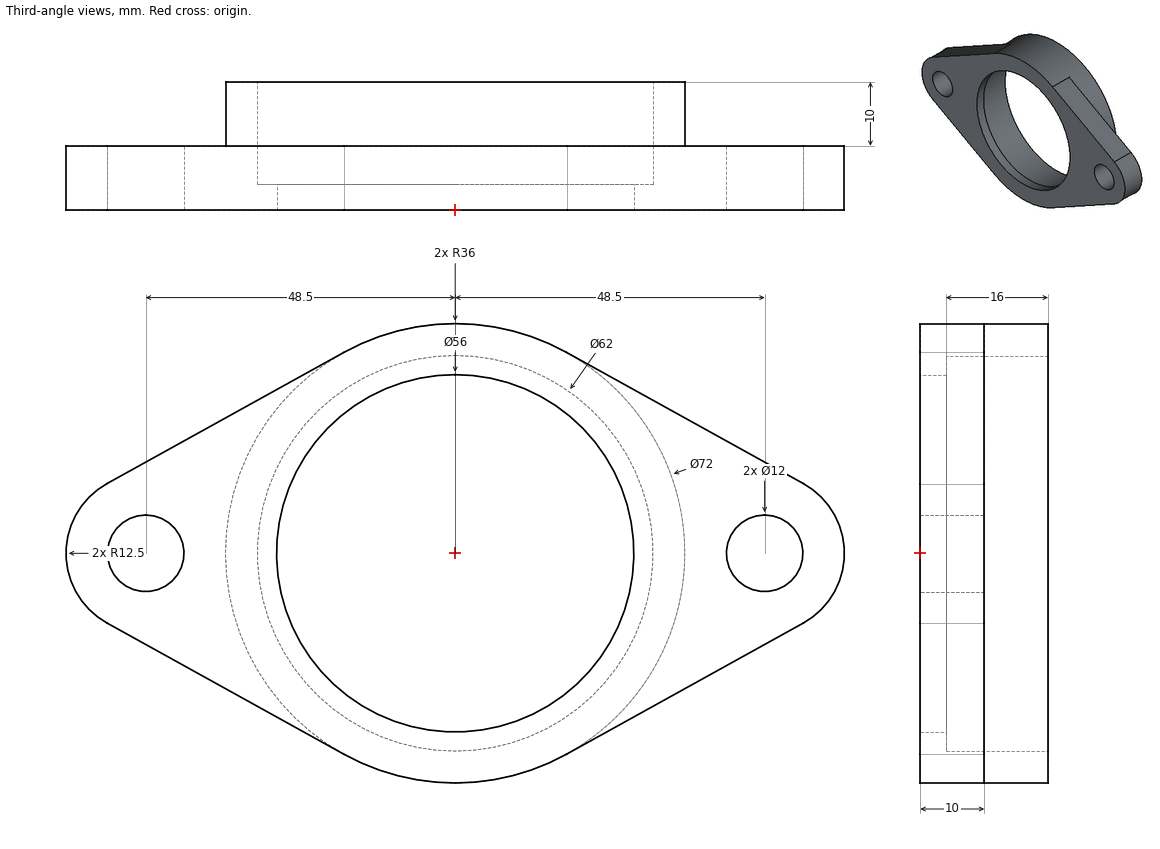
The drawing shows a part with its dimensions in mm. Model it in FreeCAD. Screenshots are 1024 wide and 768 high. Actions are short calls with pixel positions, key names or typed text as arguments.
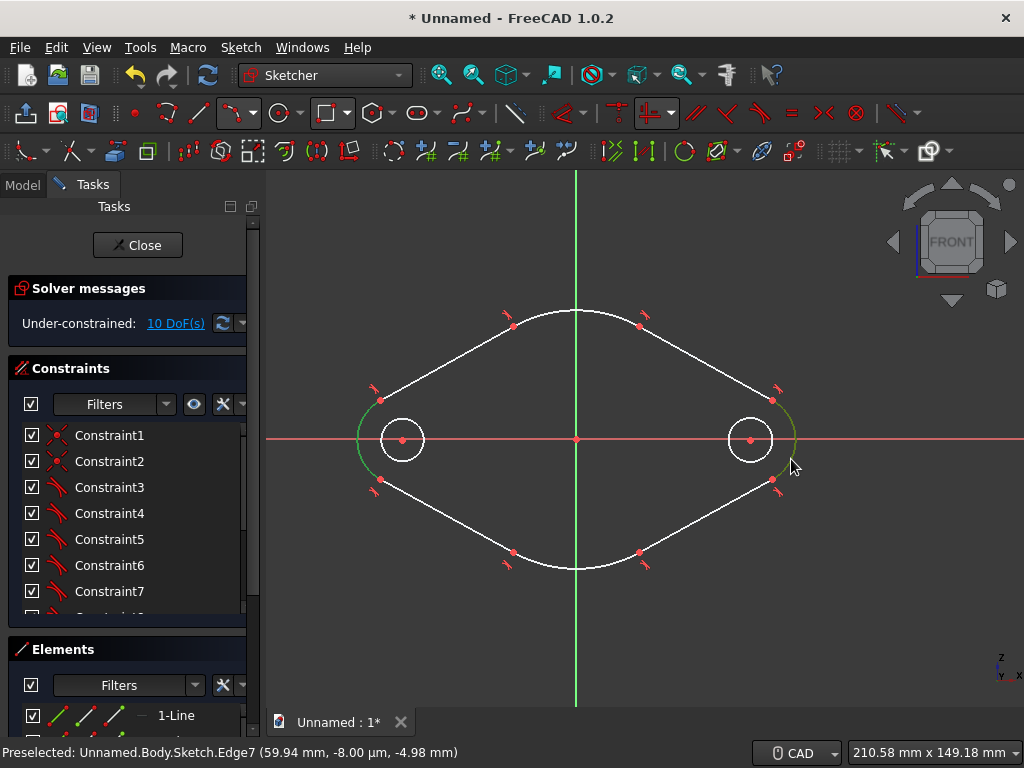
click(792, 114)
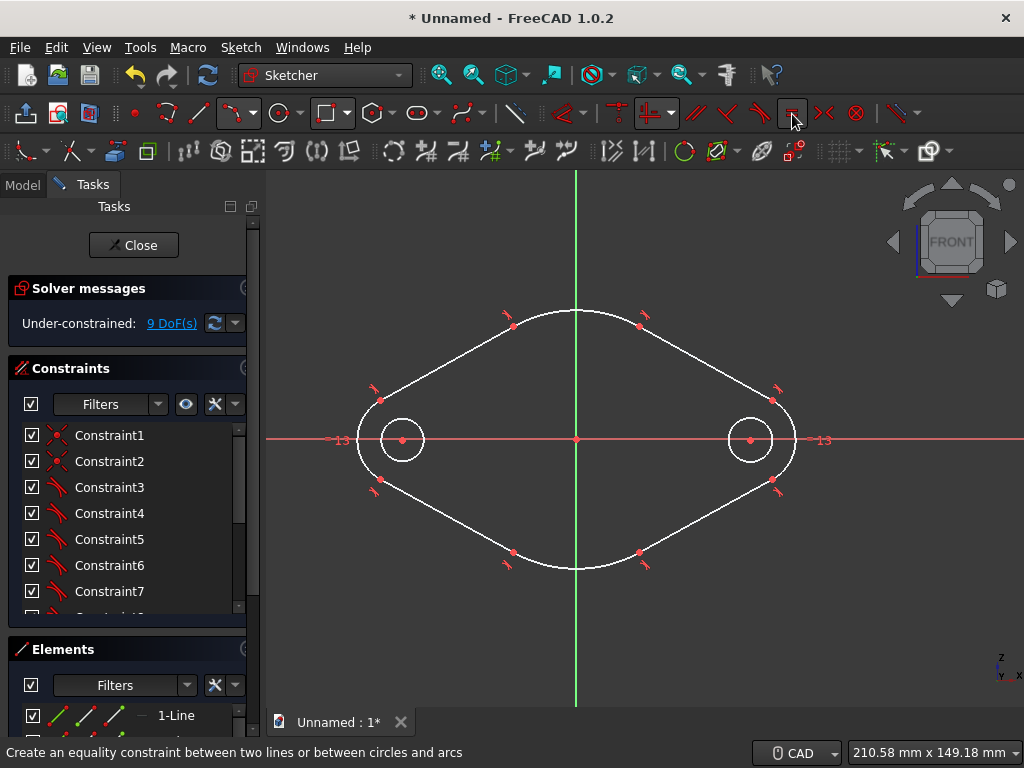
click(602, 313)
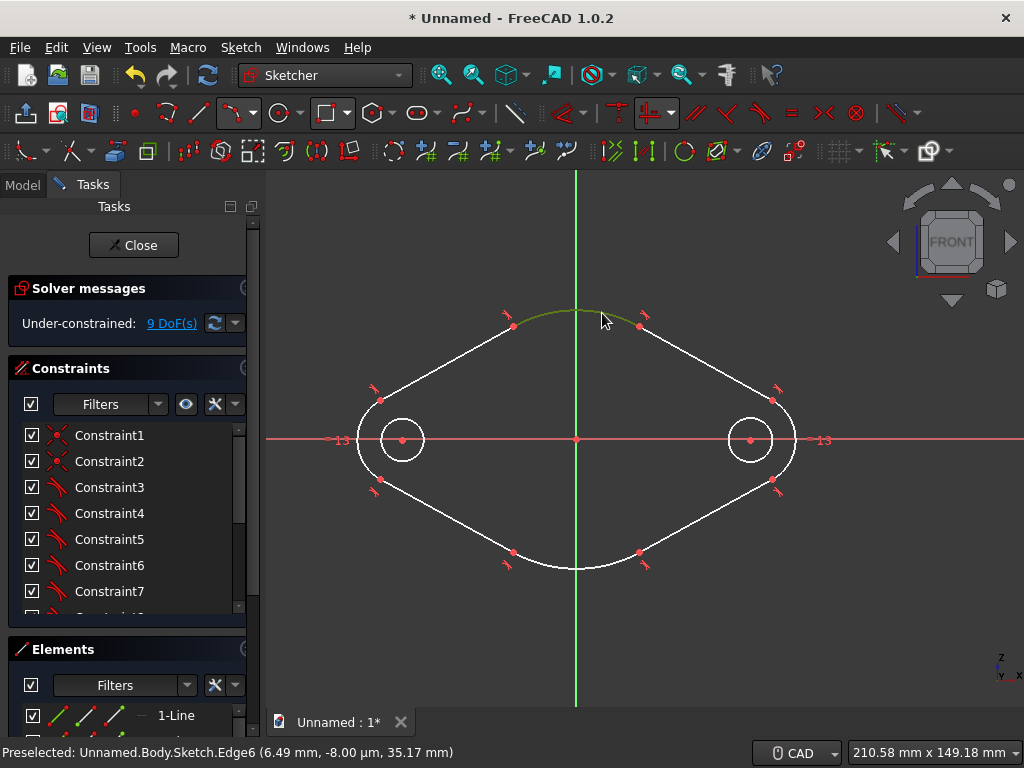
click(551, 566)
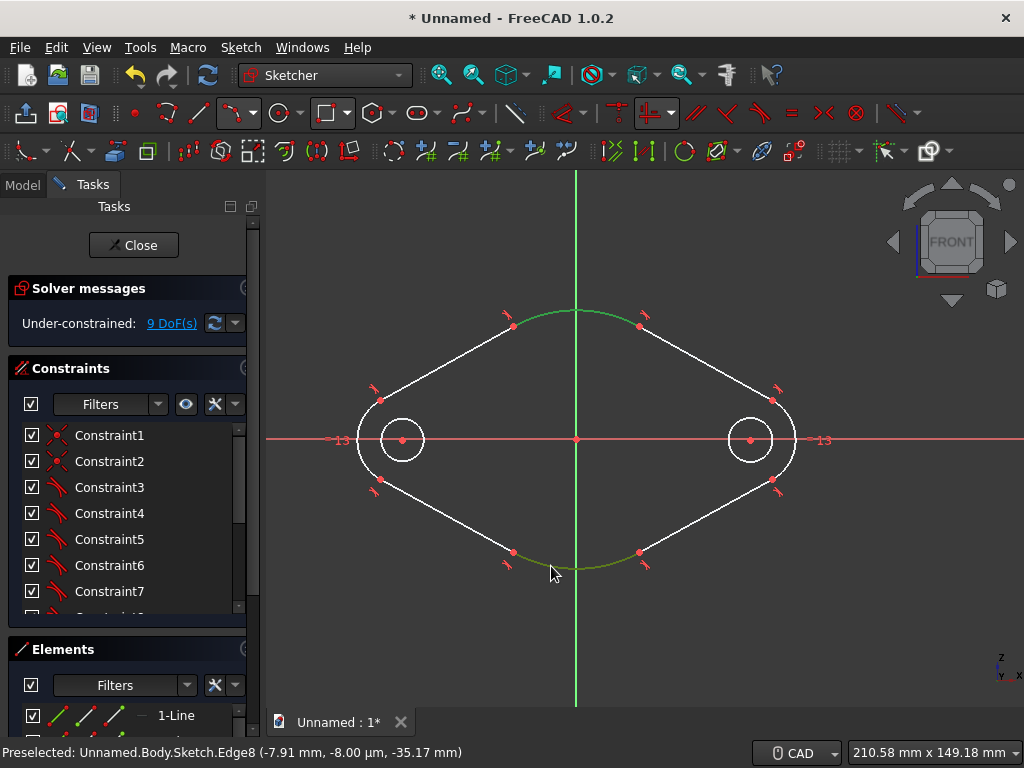
click(792, 114)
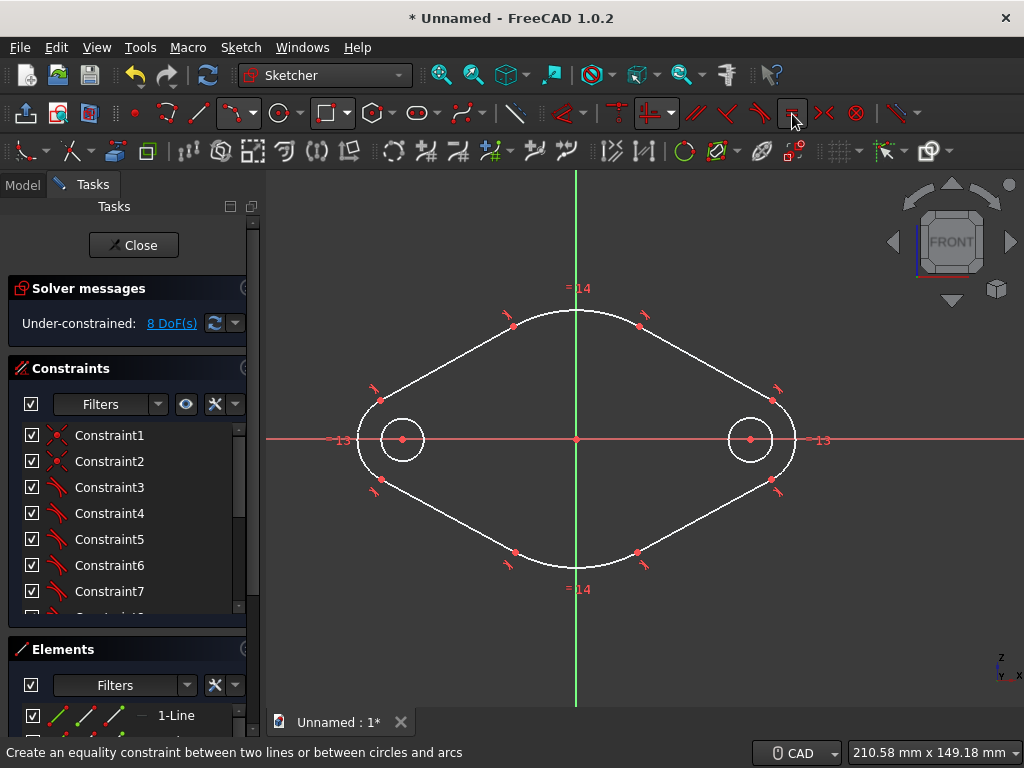
click(766, 424)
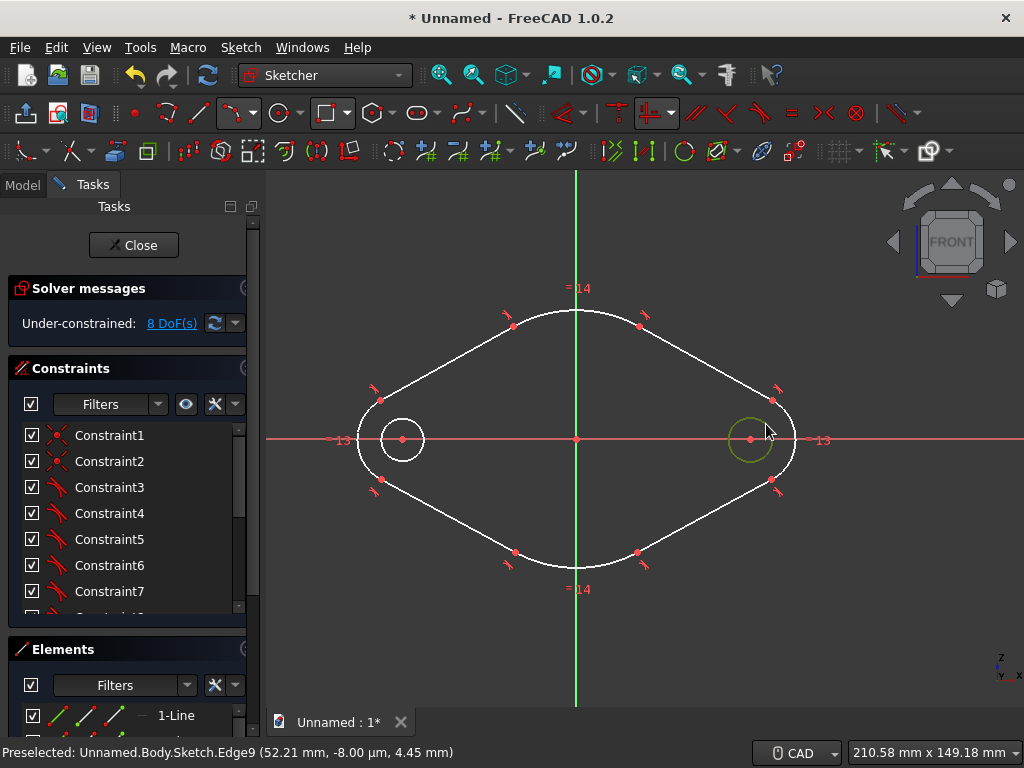
click(417, 425)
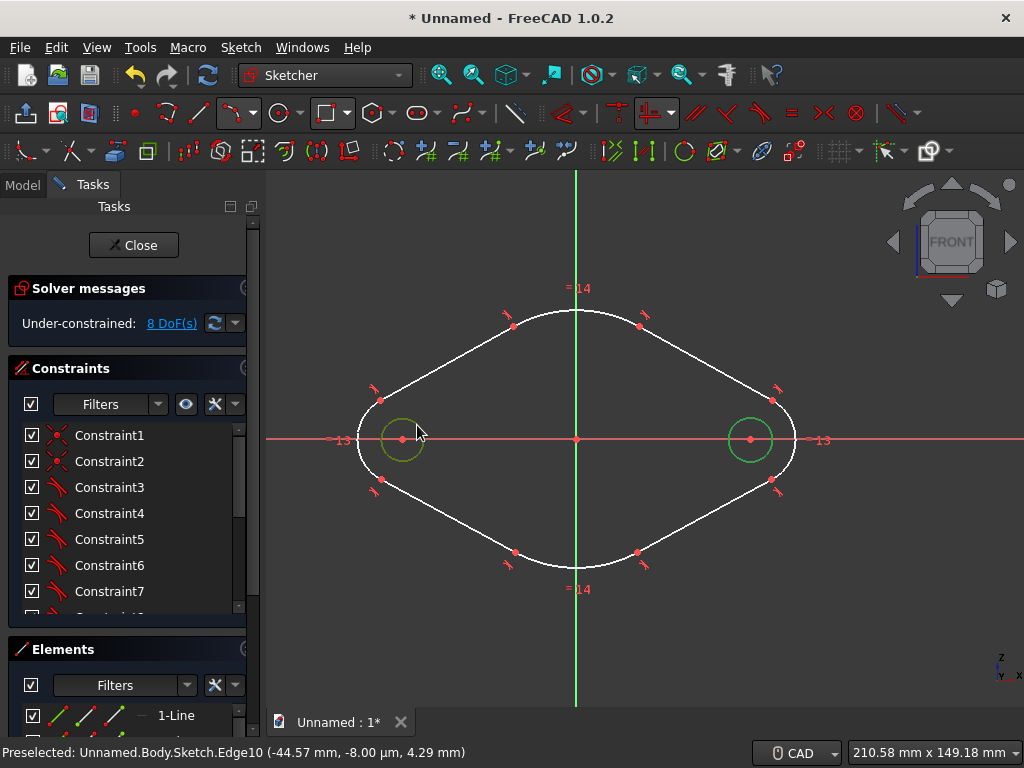
click(792, 114)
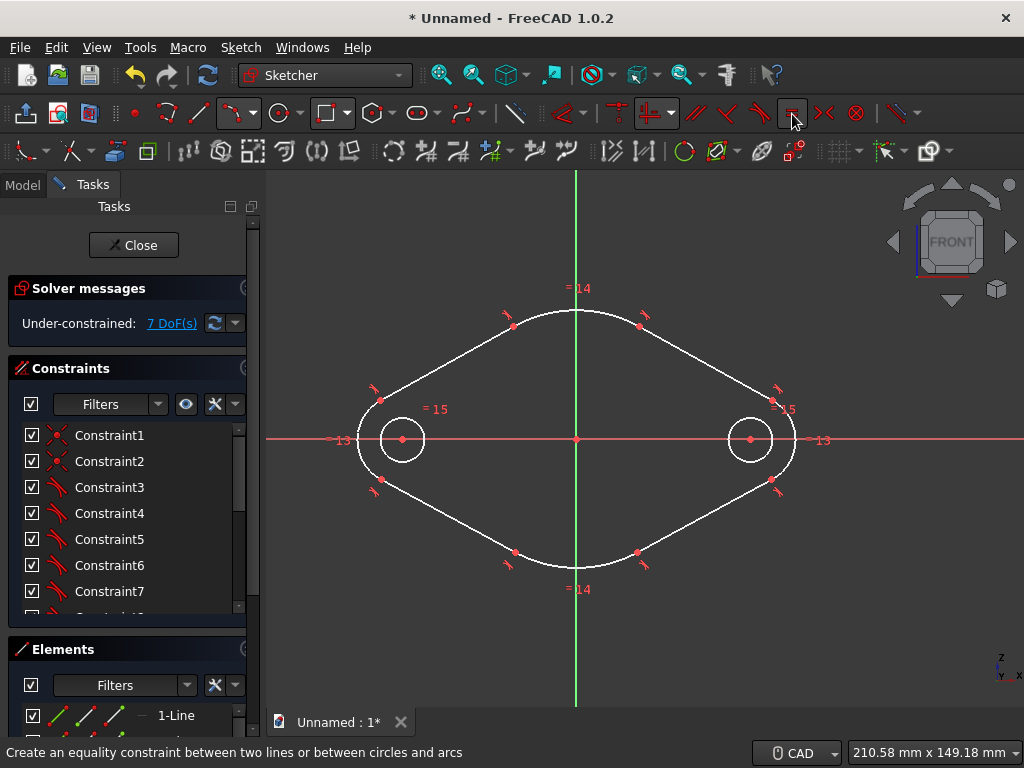
click(403, 440)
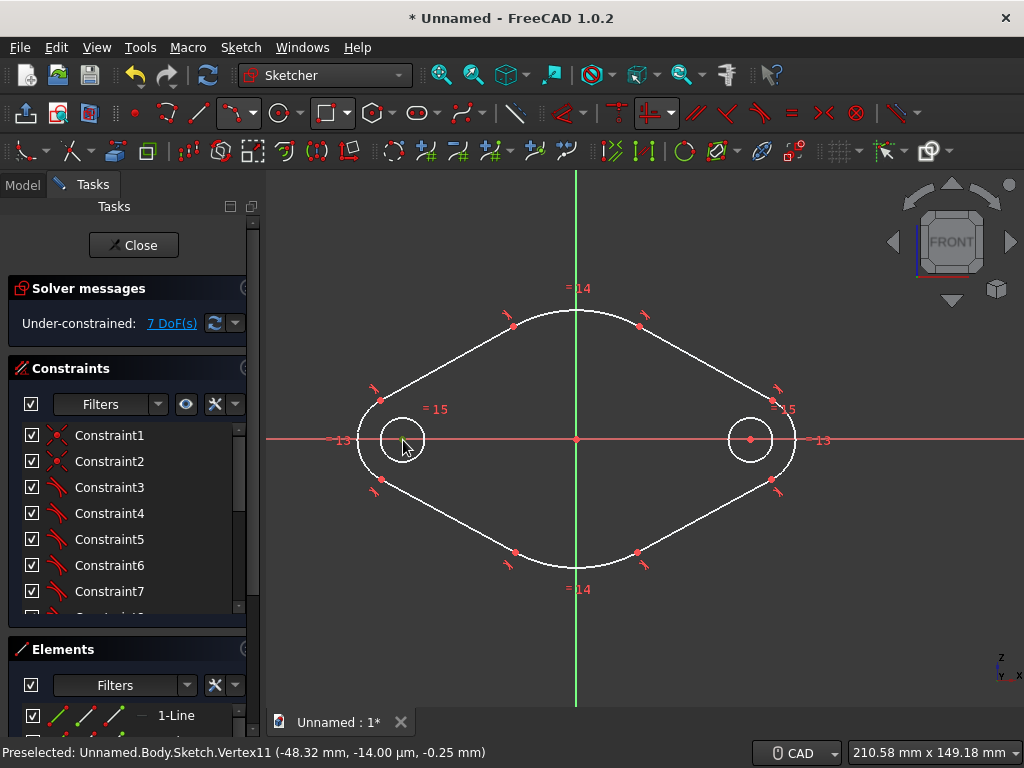
click(455, 439)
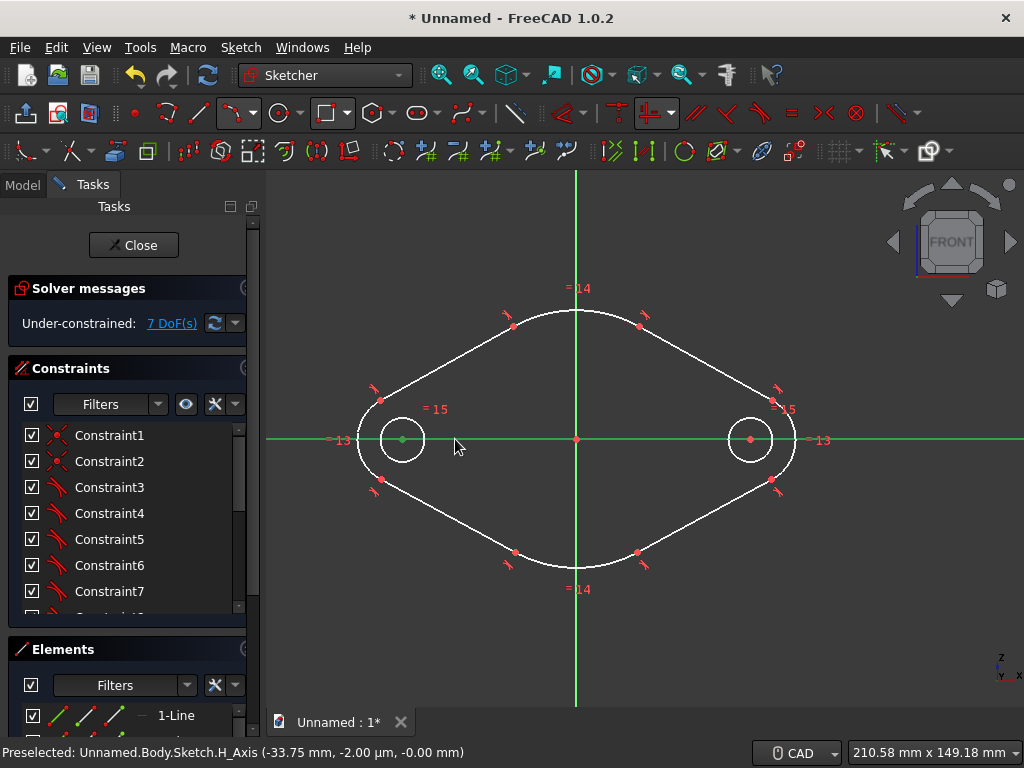
click(618, 114)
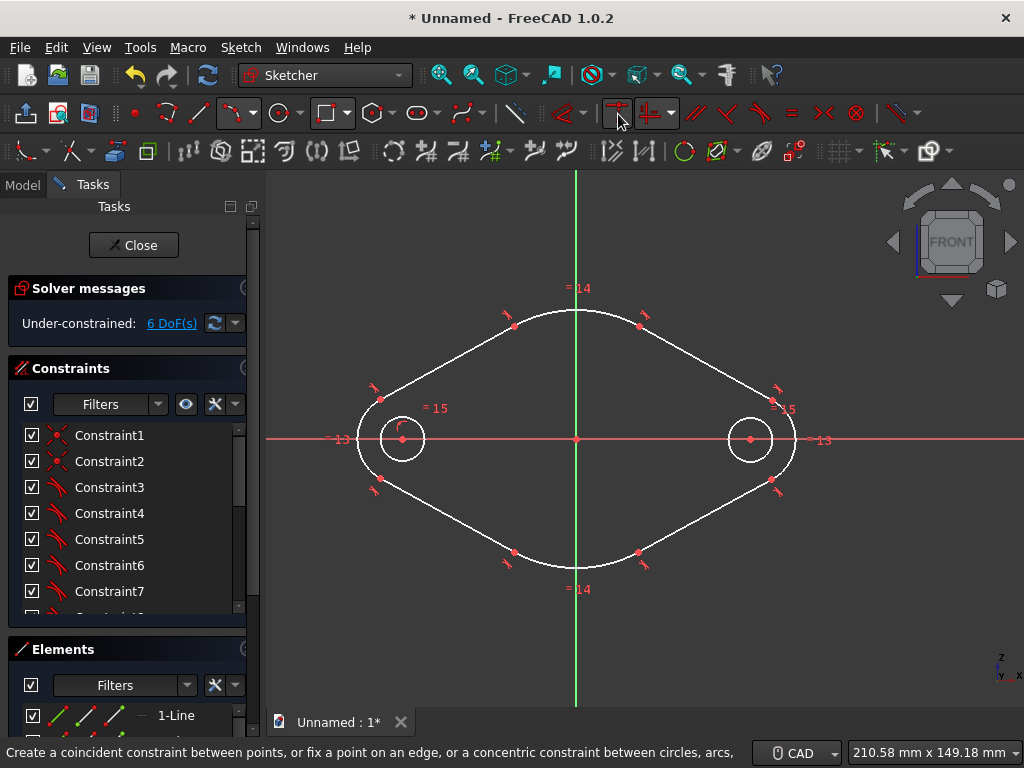
click(750, 440)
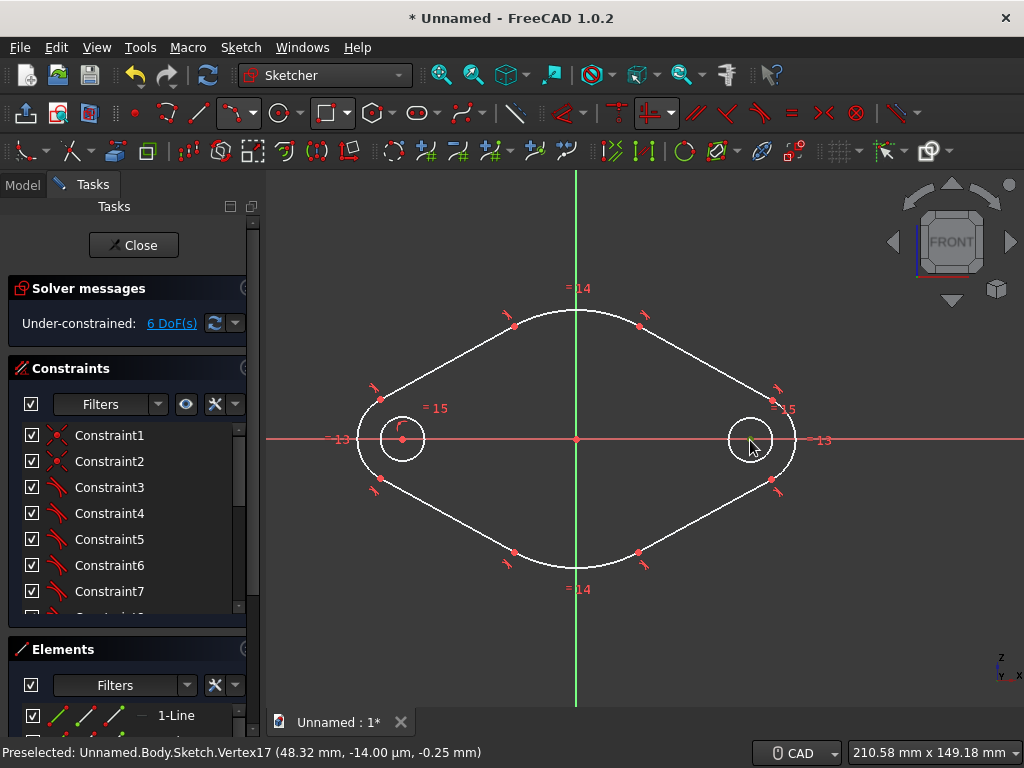
click(455, 439)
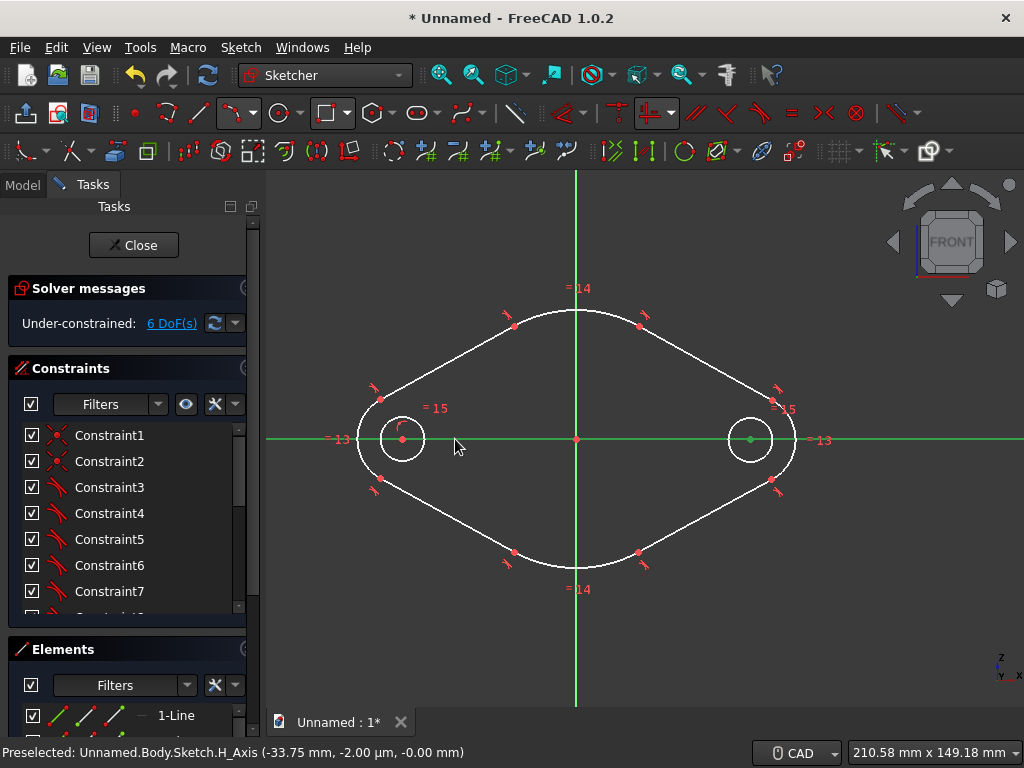
click(618, 114)